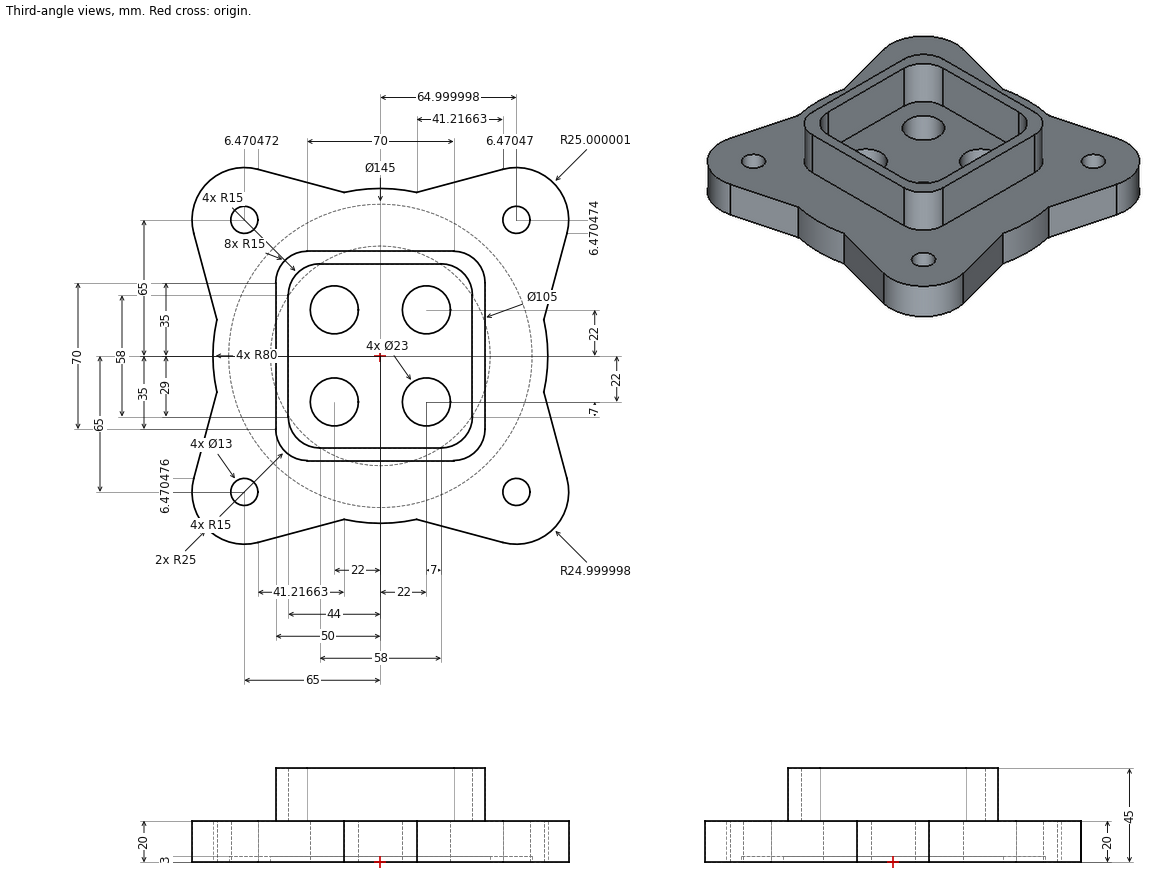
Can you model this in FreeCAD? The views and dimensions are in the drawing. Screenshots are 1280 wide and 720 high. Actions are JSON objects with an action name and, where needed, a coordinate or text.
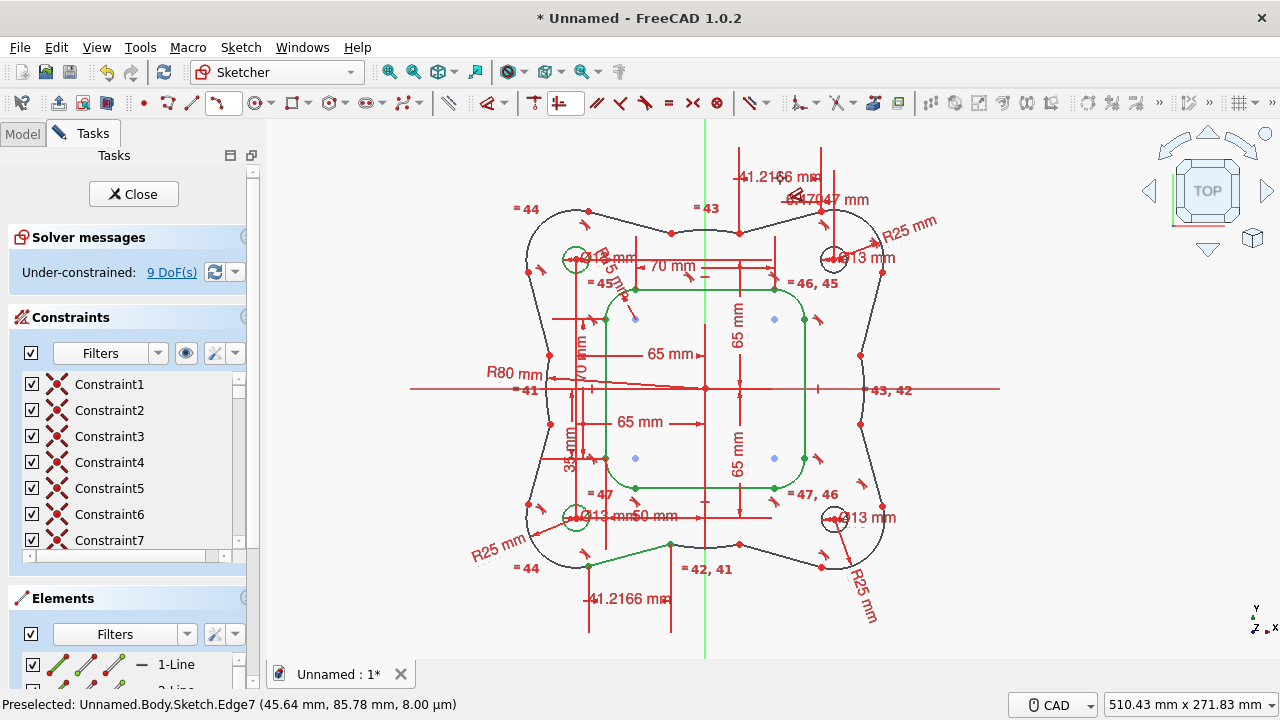
{"action": "left_click", "coordinate": [835, 520]}
{"action": "left_click", "coordinate": [770, 355]}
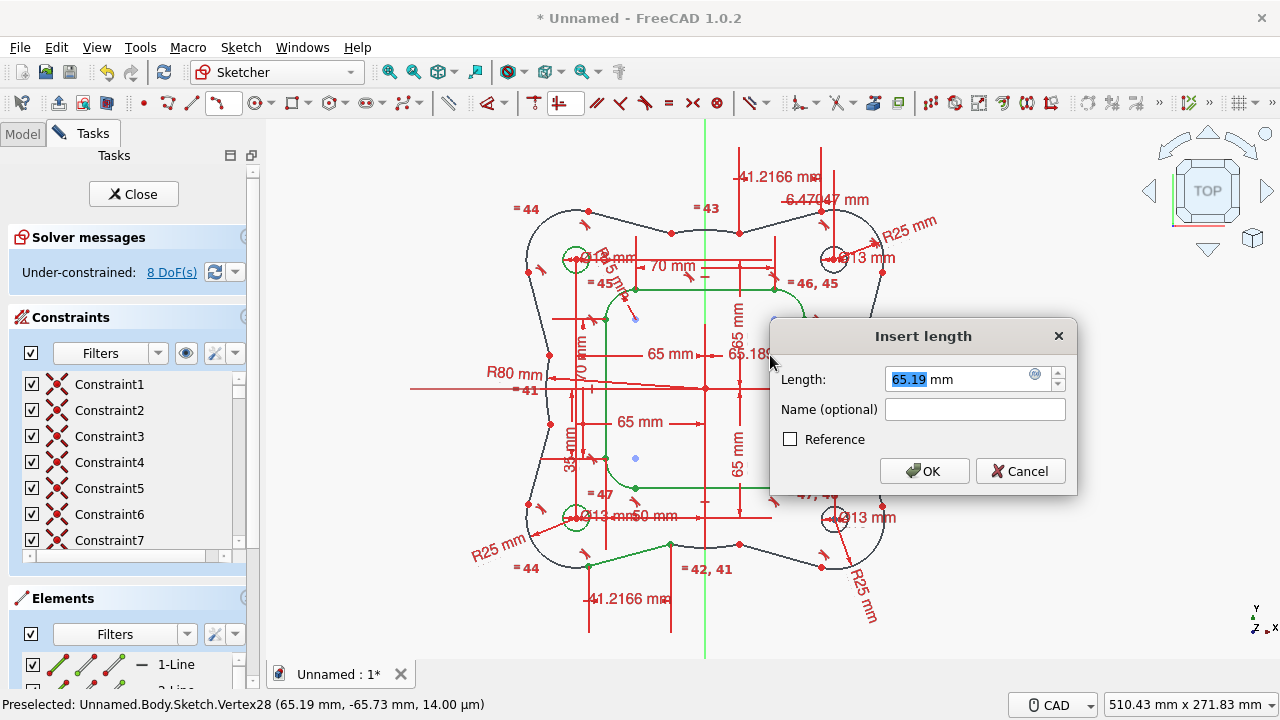
{"action": "type", "text": "65.000003"}
{"action": "key", "text": "Return"}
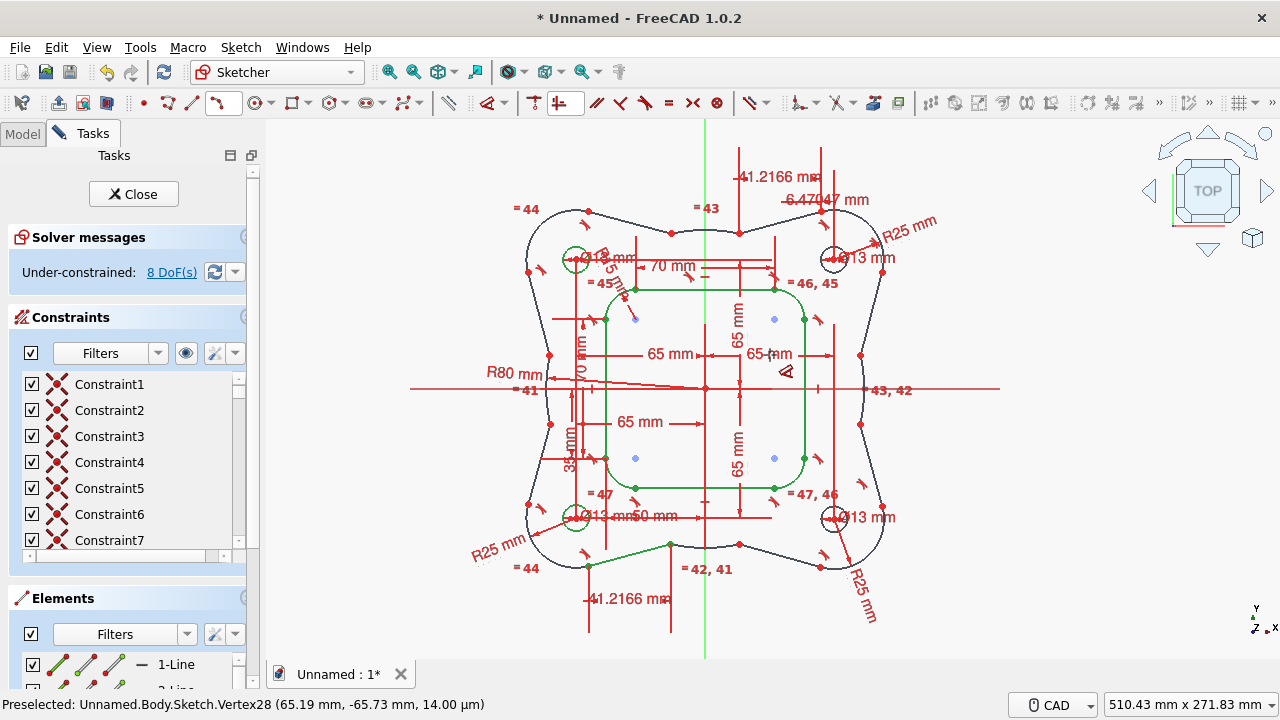
{"action": "left_click", "coordinate": [834, 519]}
{"action": "left_click", "coordinate": [892, 454]}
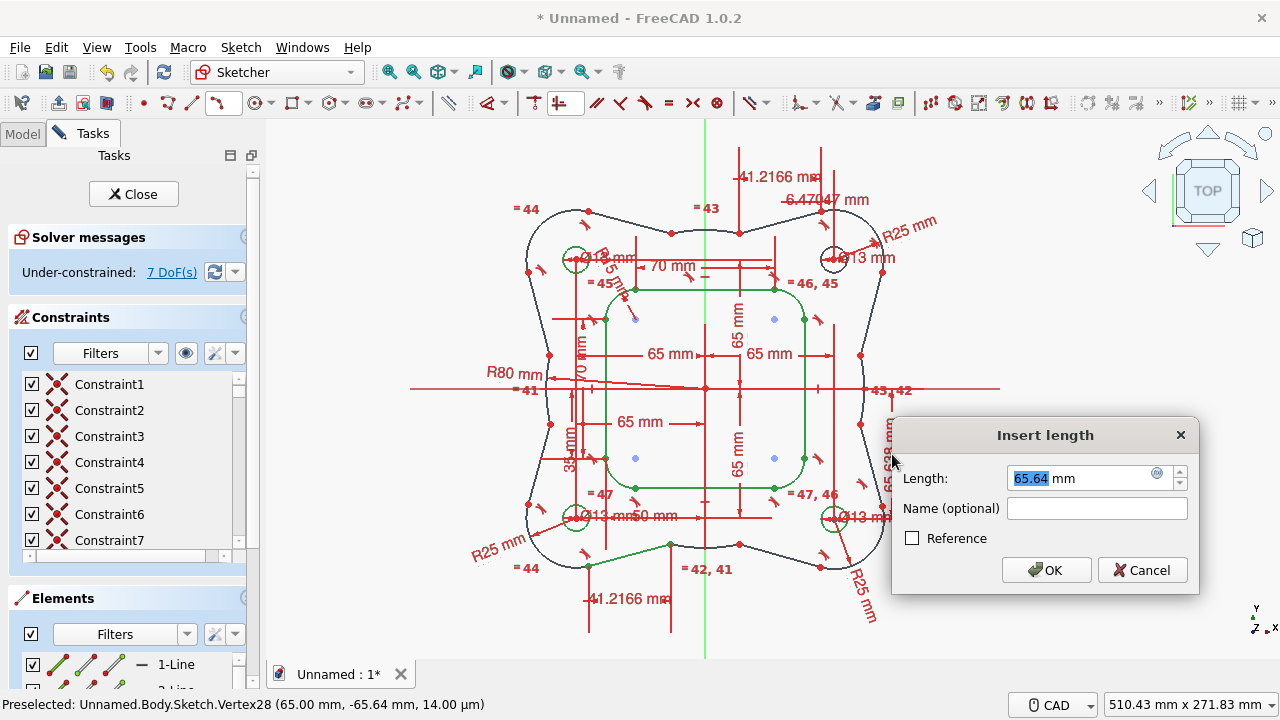
{"action": "type", "text": "65.000003"}
{"action": "key", "text": "Return"}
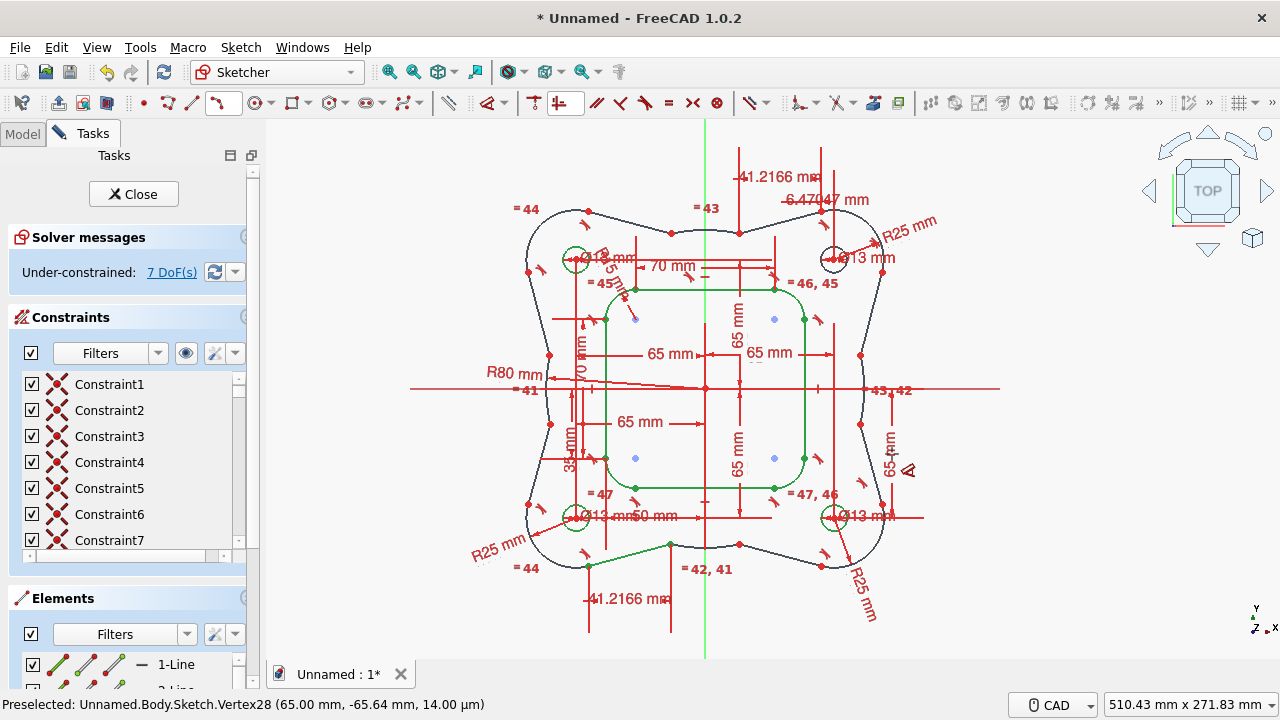
{"action": "left_click", "coordinate": [834, 260]}
{"action": "left_click", "coordinate": [770, 423]}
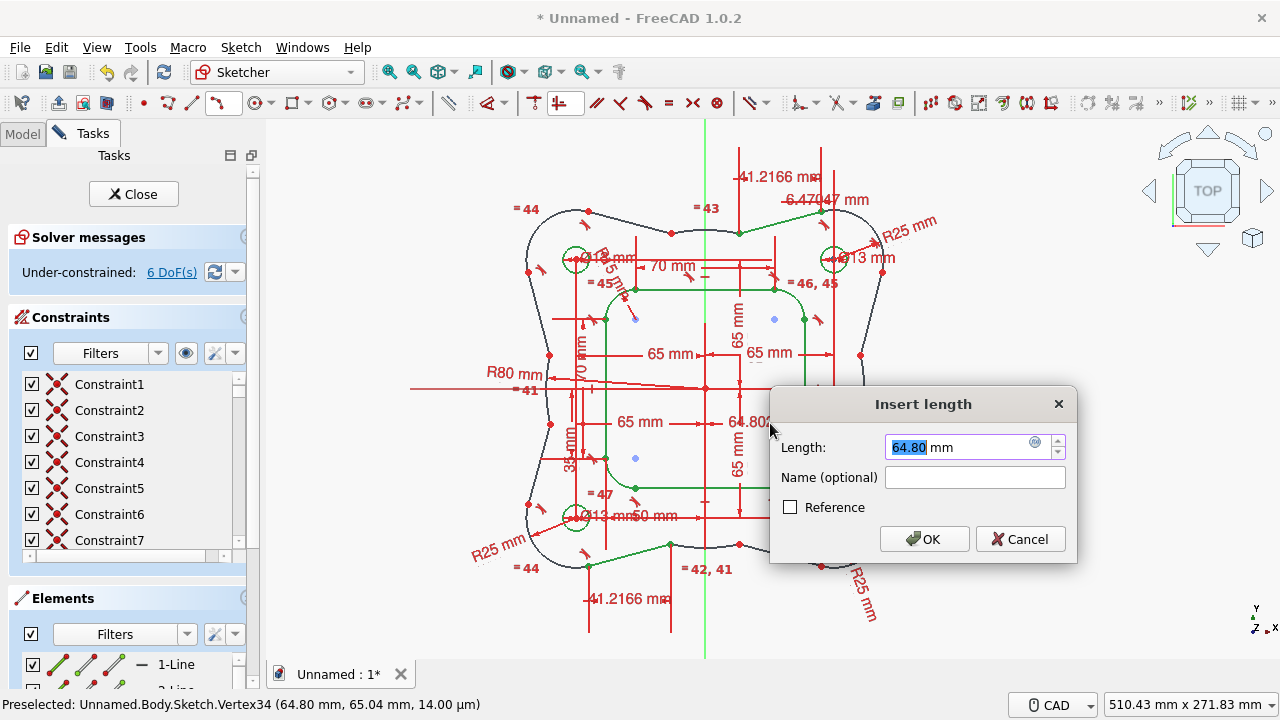
{"action": "type", "text": "64.999998"}
{"action": "key", "text": "Return"}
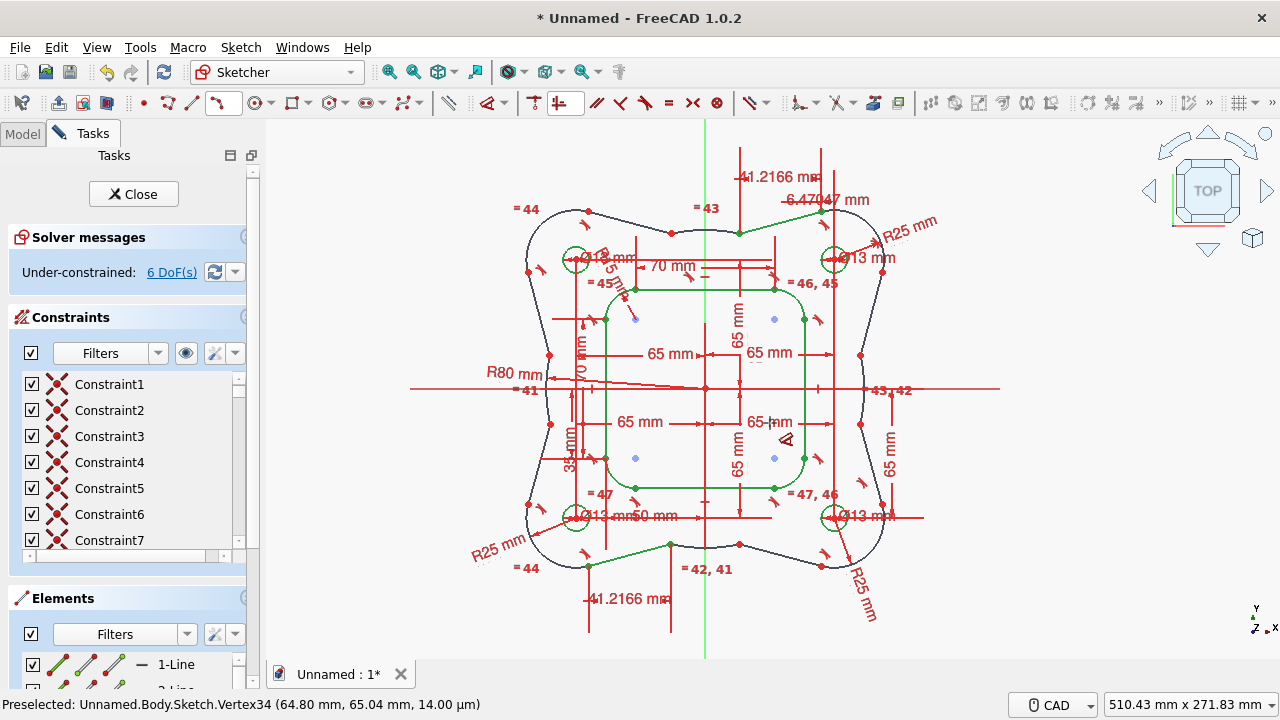
{"action": "scroll", "coordinate": [528, 505], "scroll_direction": "up", "scroll_amount": 6}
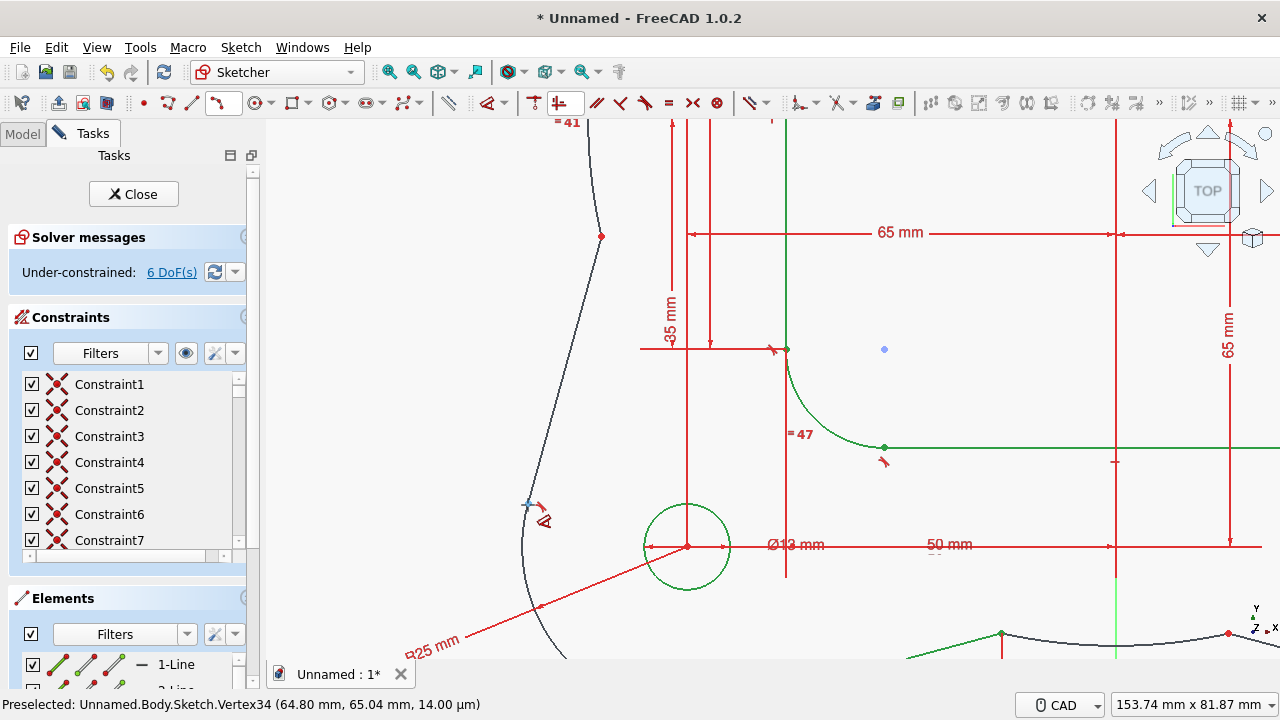
{"action": "left_click", "coordinate": [528, 503]}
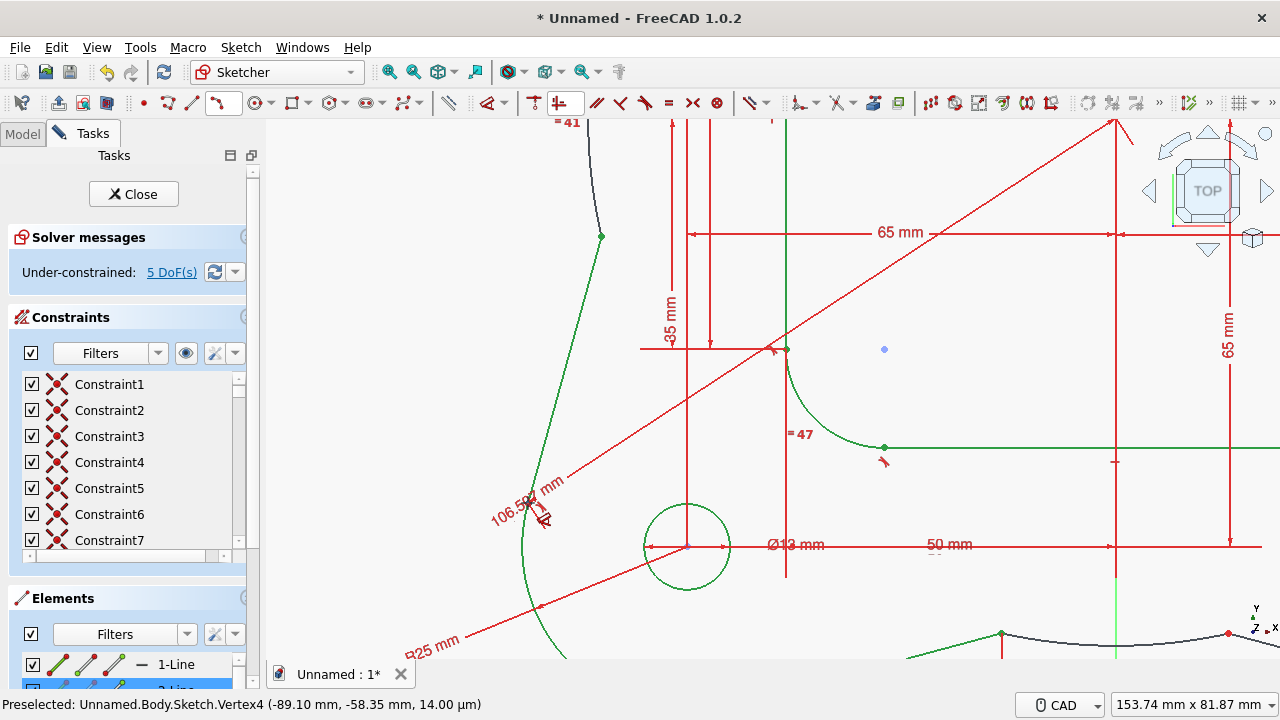
{"action": "left_click", "coordinate": [687, 547]}
{"action": "left_click", "coordinate": [494, 525]}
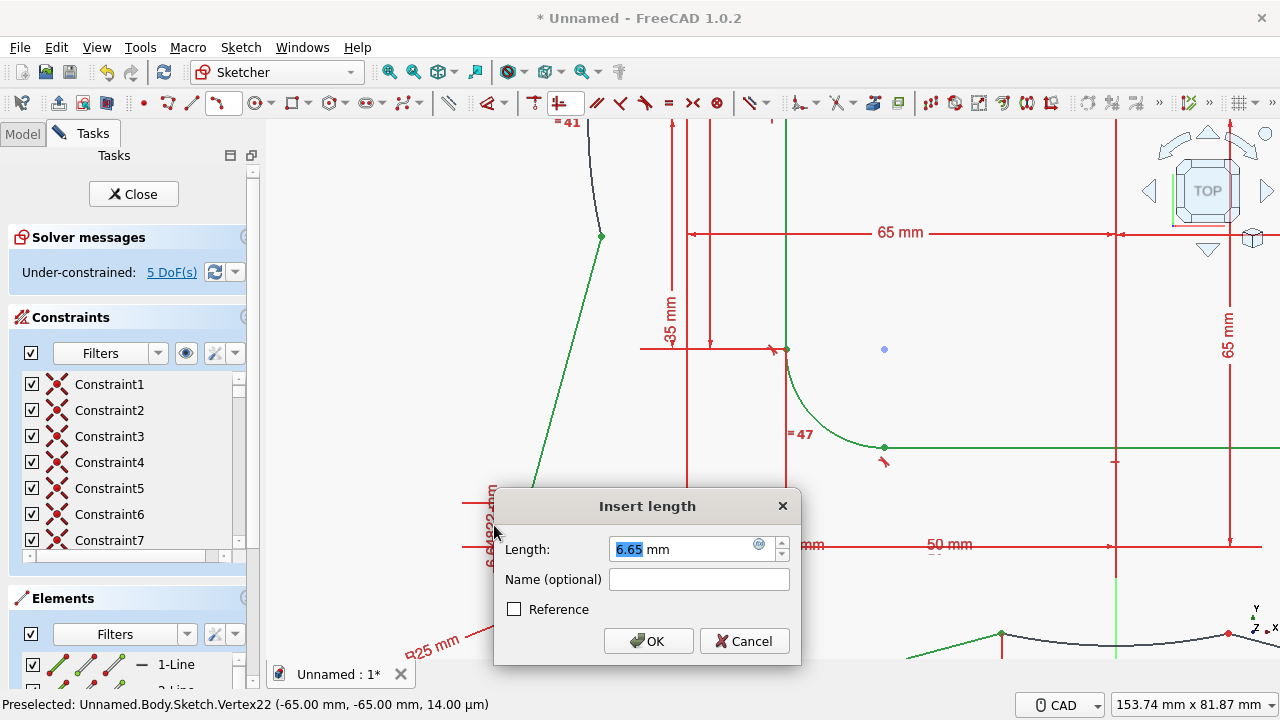
{"action": "type", "text": "6.470476"}
{"action": "key", "text": "Return"}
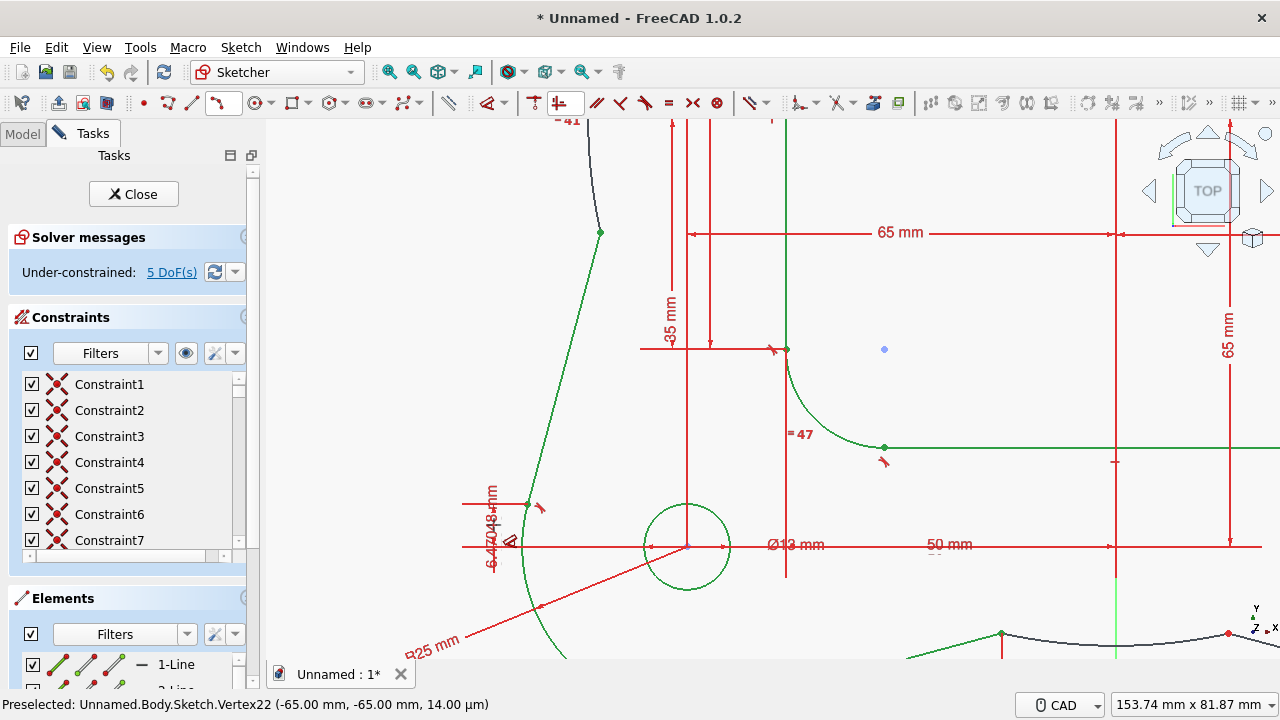
{"action": "scroll", "coordinate": [527, 506], "scroll_direction": "down", "scroll_amount": 6}